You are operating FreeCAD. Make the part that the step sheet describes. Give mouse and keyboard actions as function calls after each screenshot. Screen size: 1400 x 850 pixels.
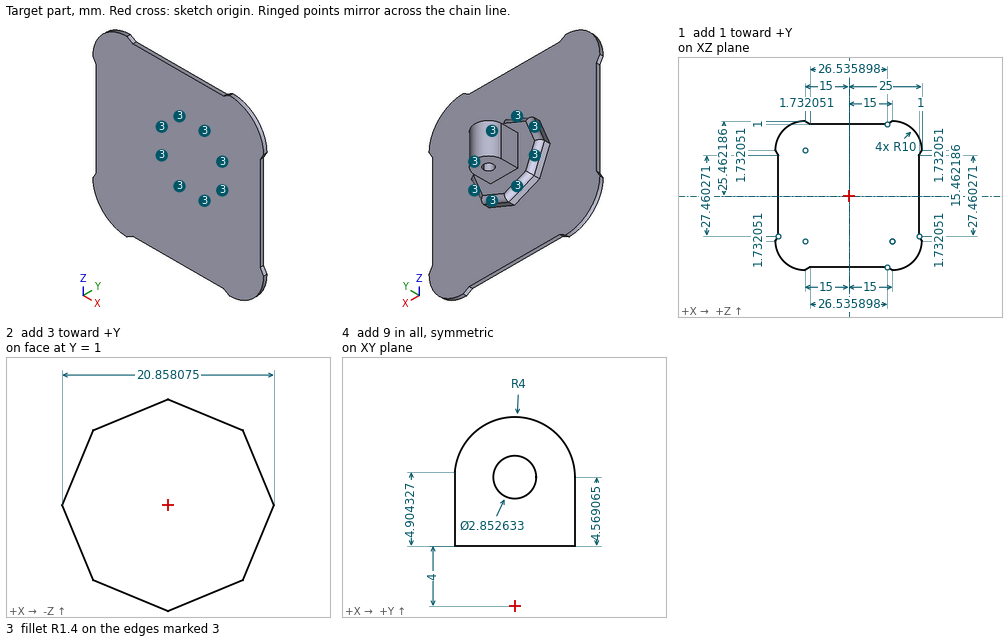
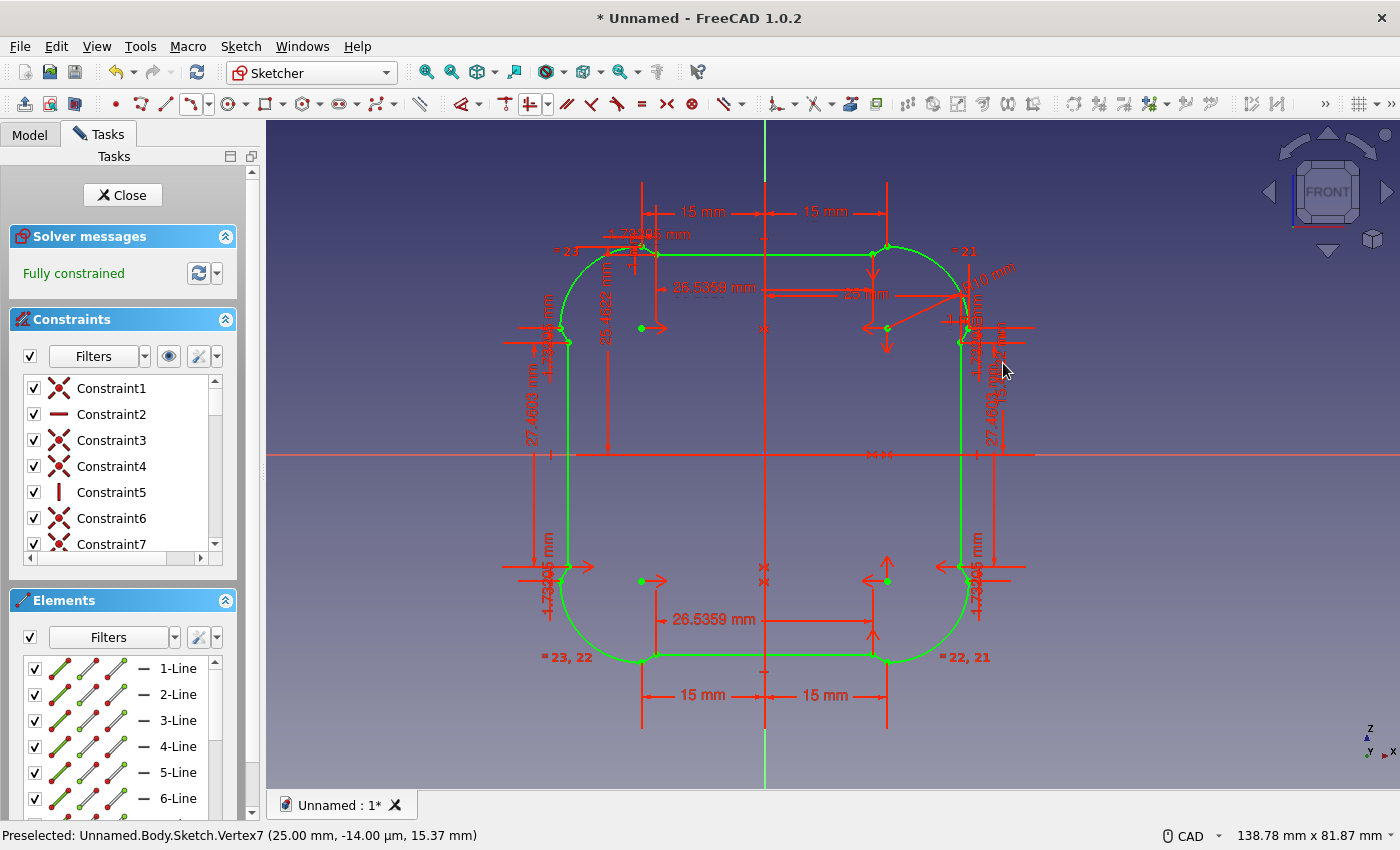
click(123, 195)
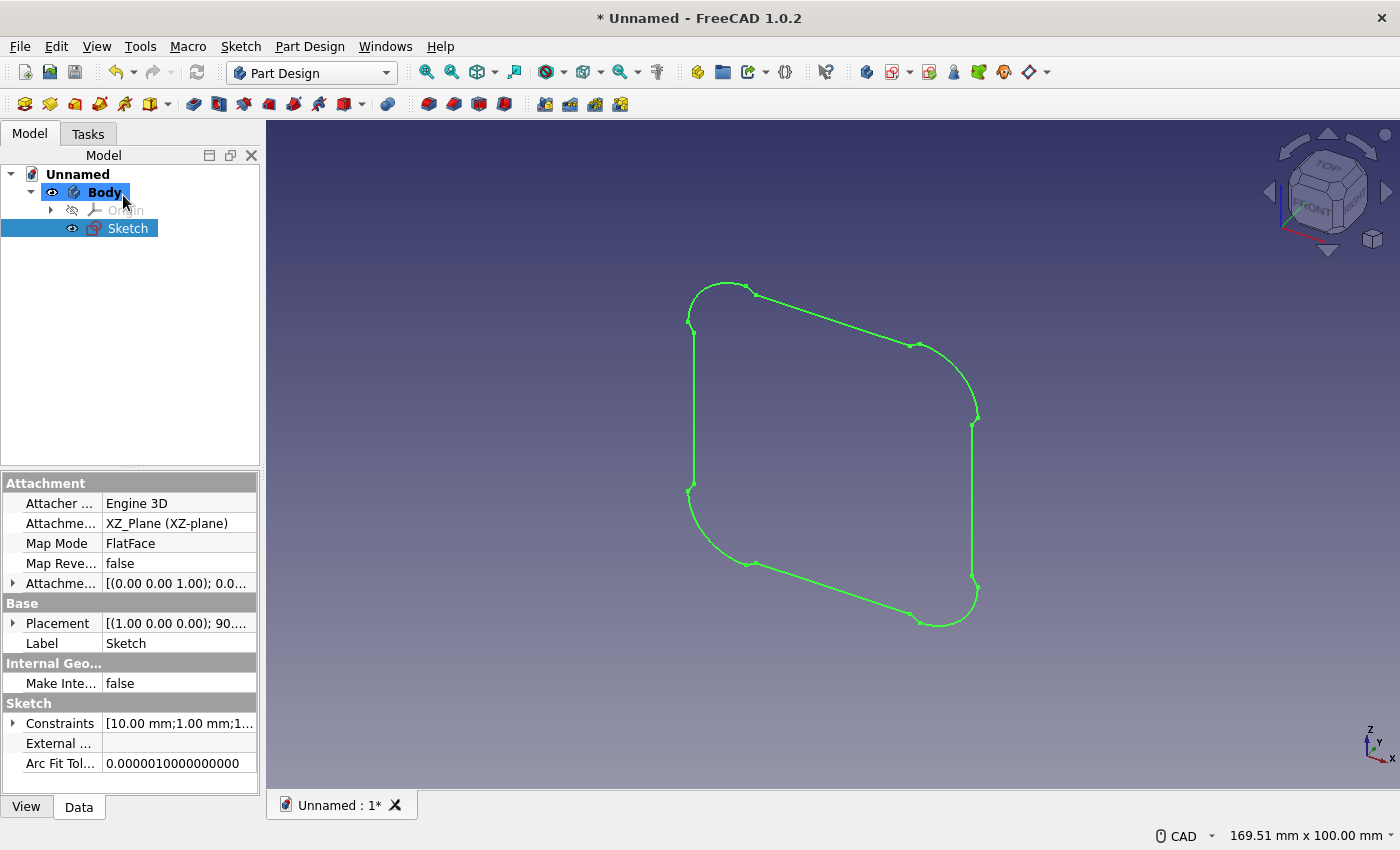
click(25, 104)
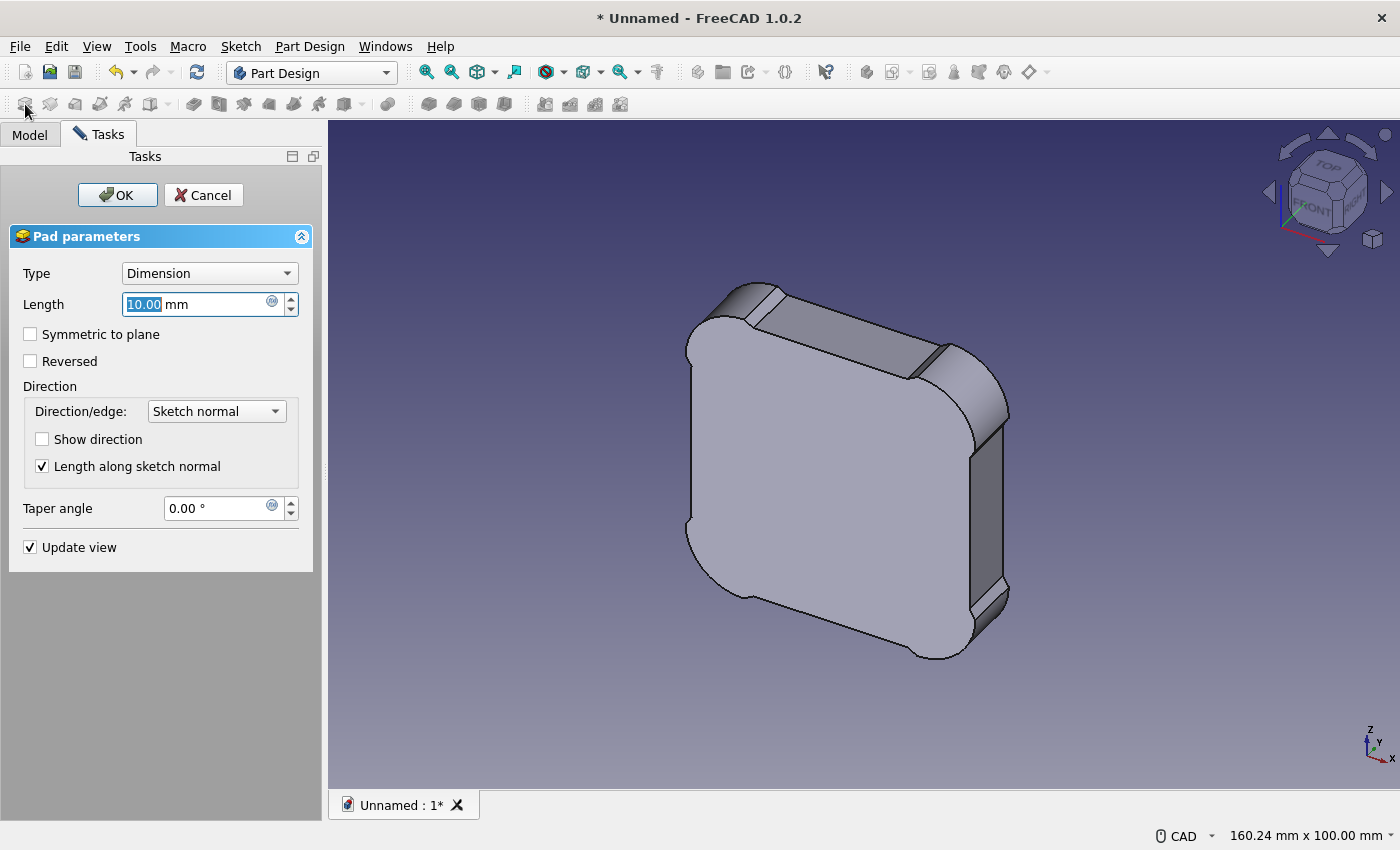
text(1)
key(Tab)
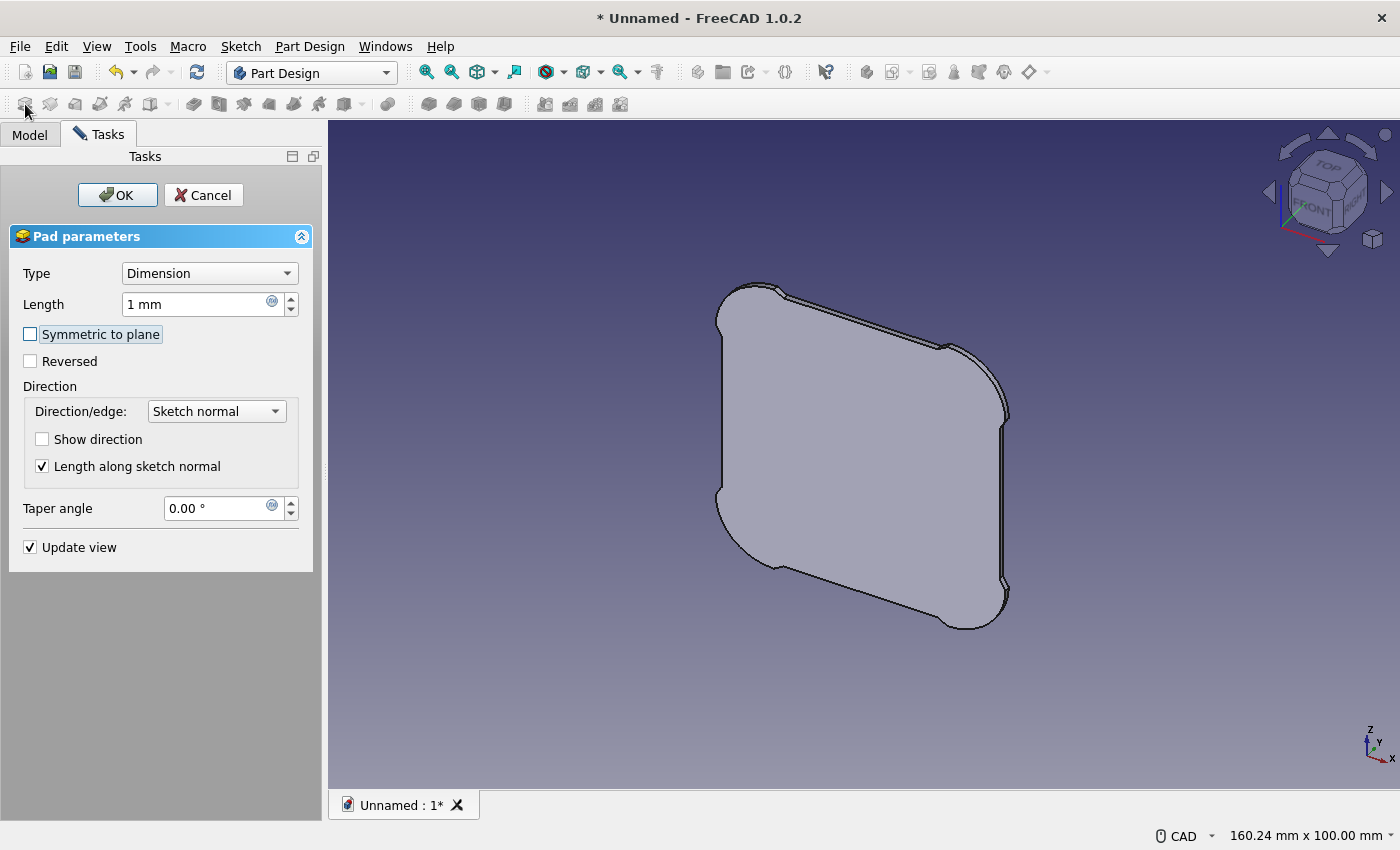
click(31, 361)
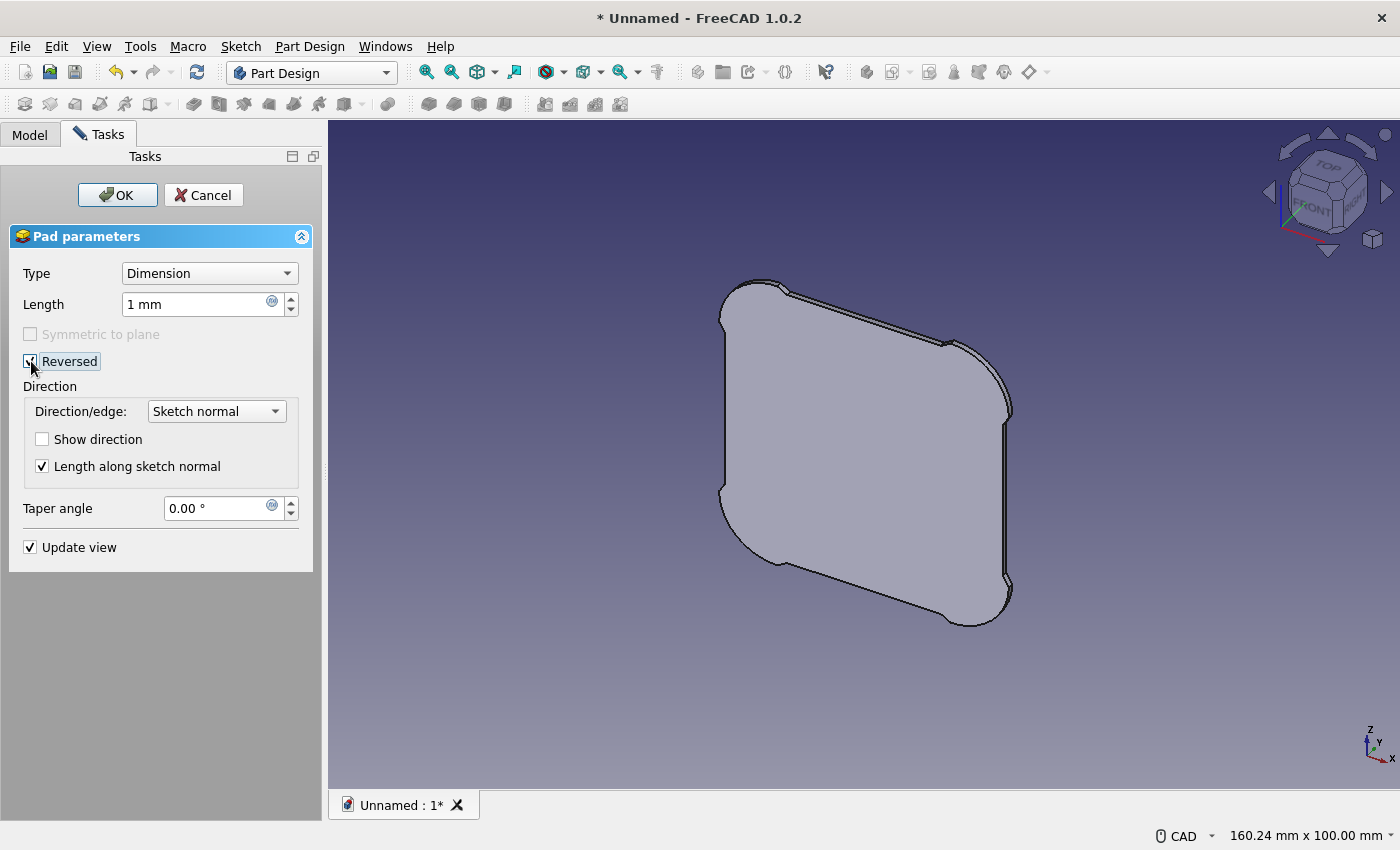
click(118, 195)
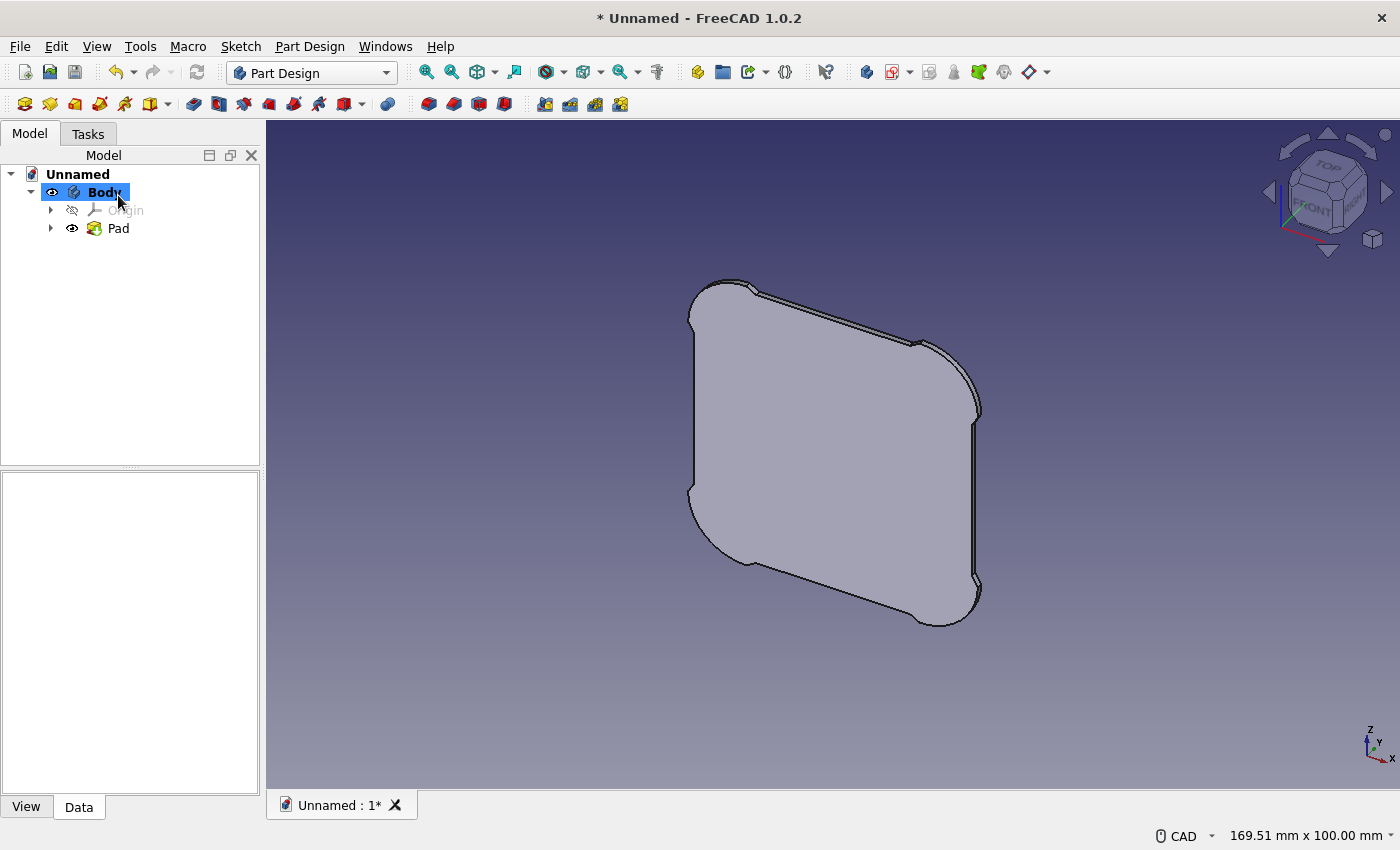
key(4)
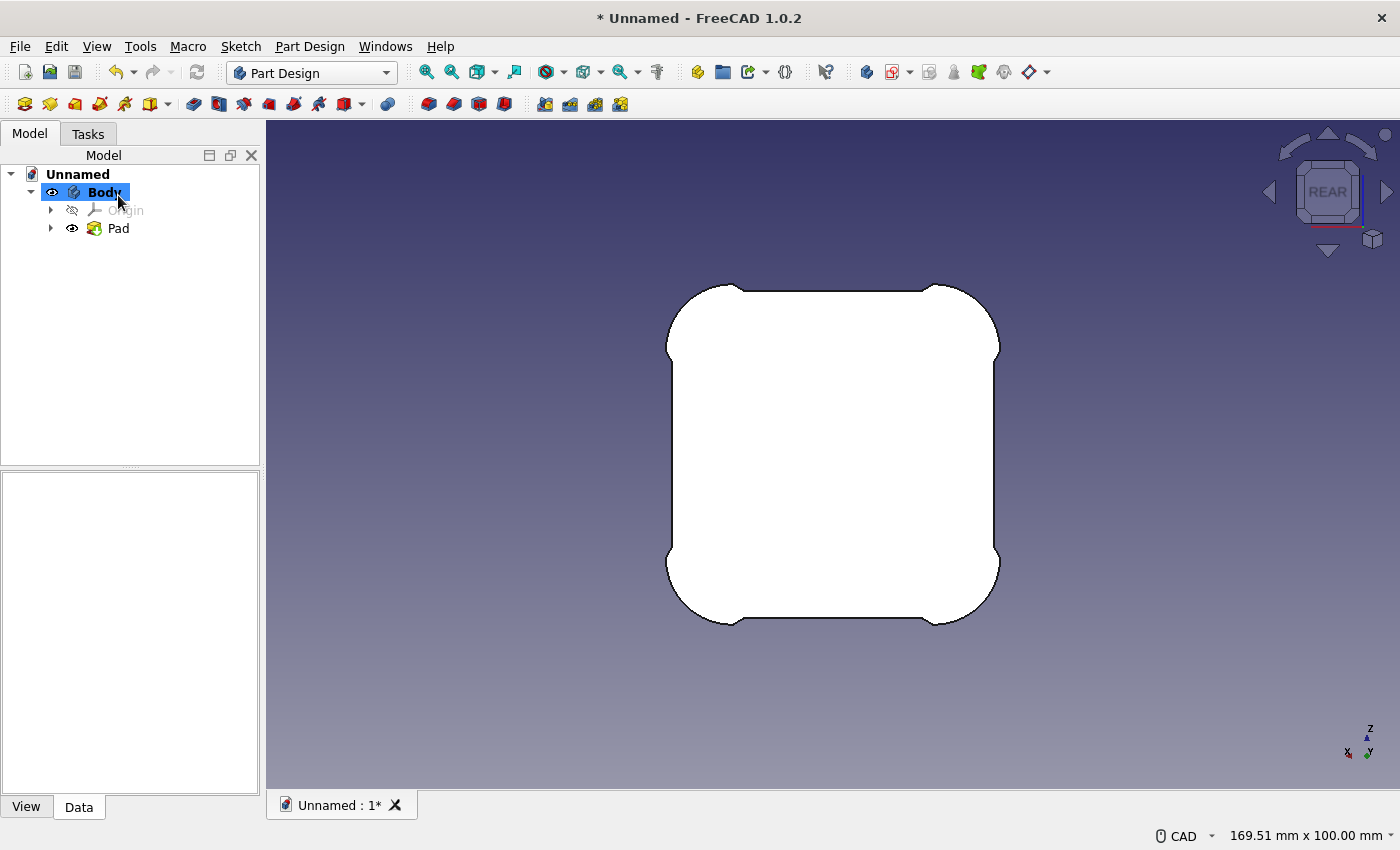
click(833, 453)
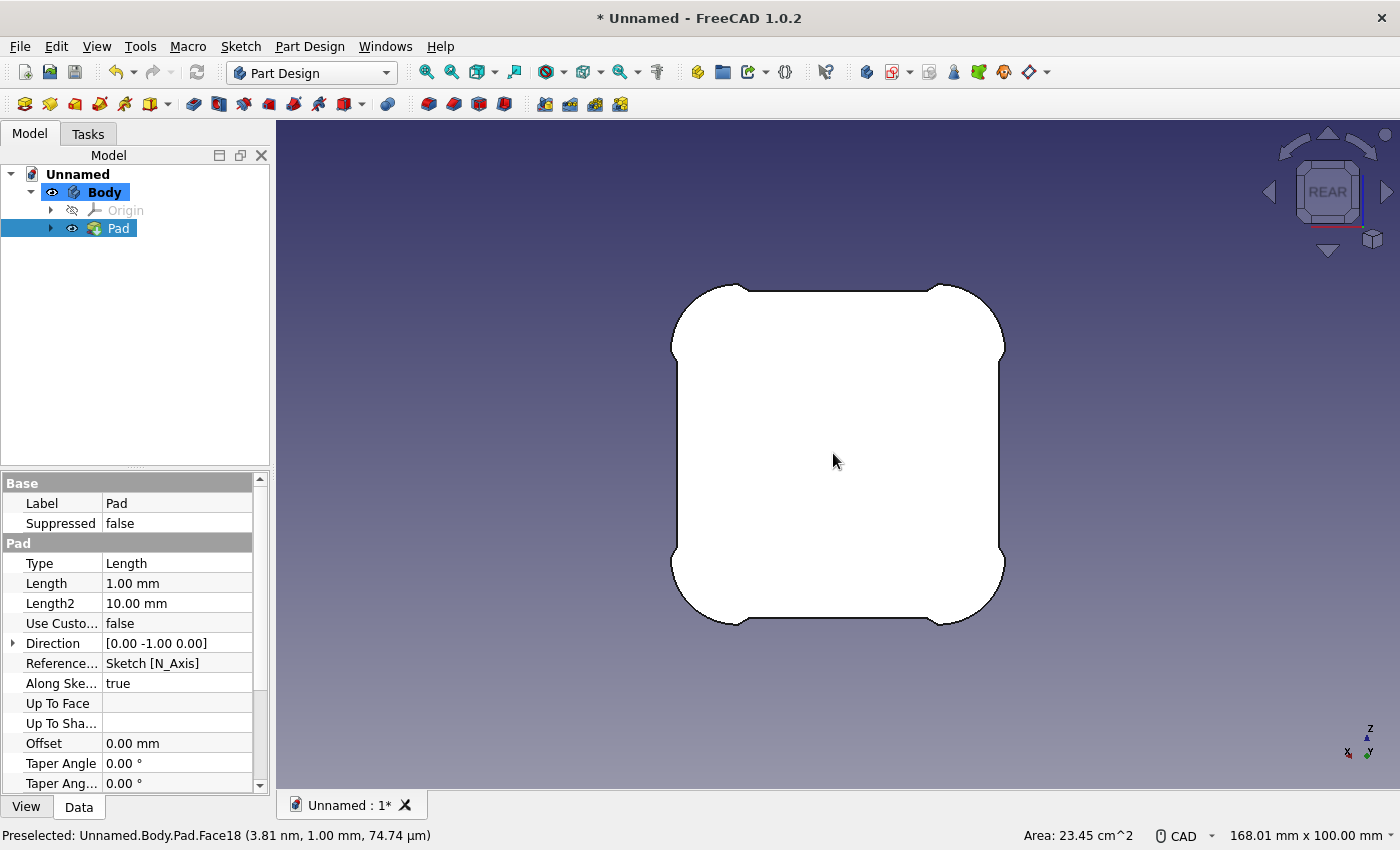
click(892, 72)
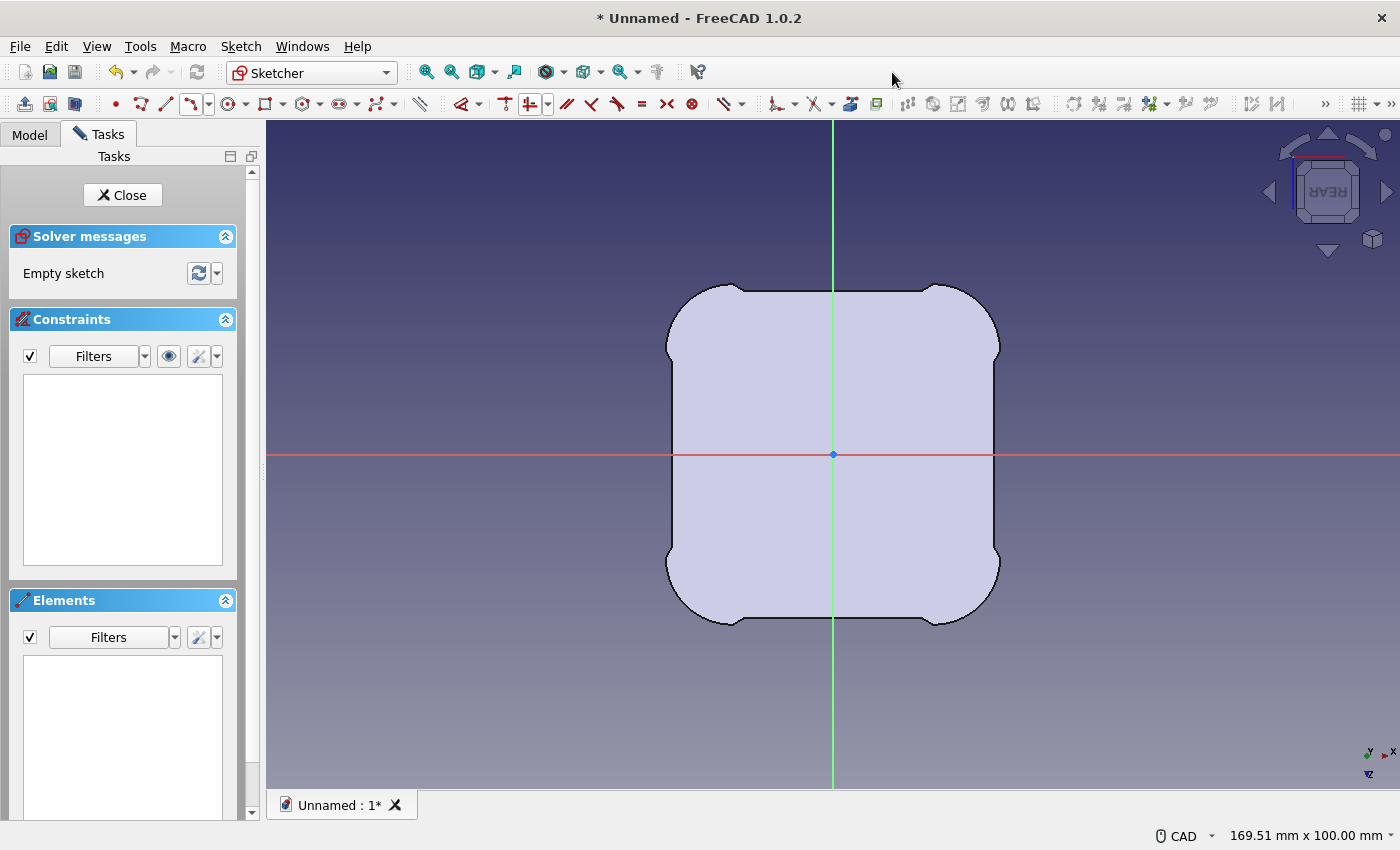
scroll(863, 455, up, 6)